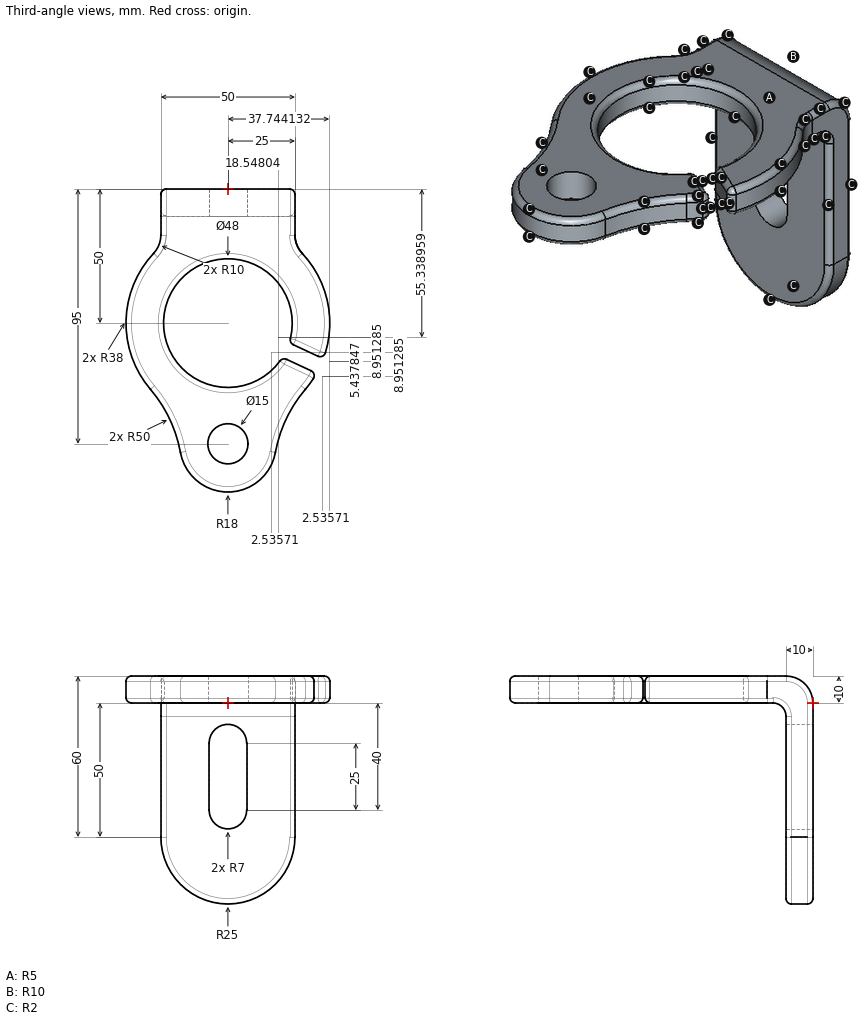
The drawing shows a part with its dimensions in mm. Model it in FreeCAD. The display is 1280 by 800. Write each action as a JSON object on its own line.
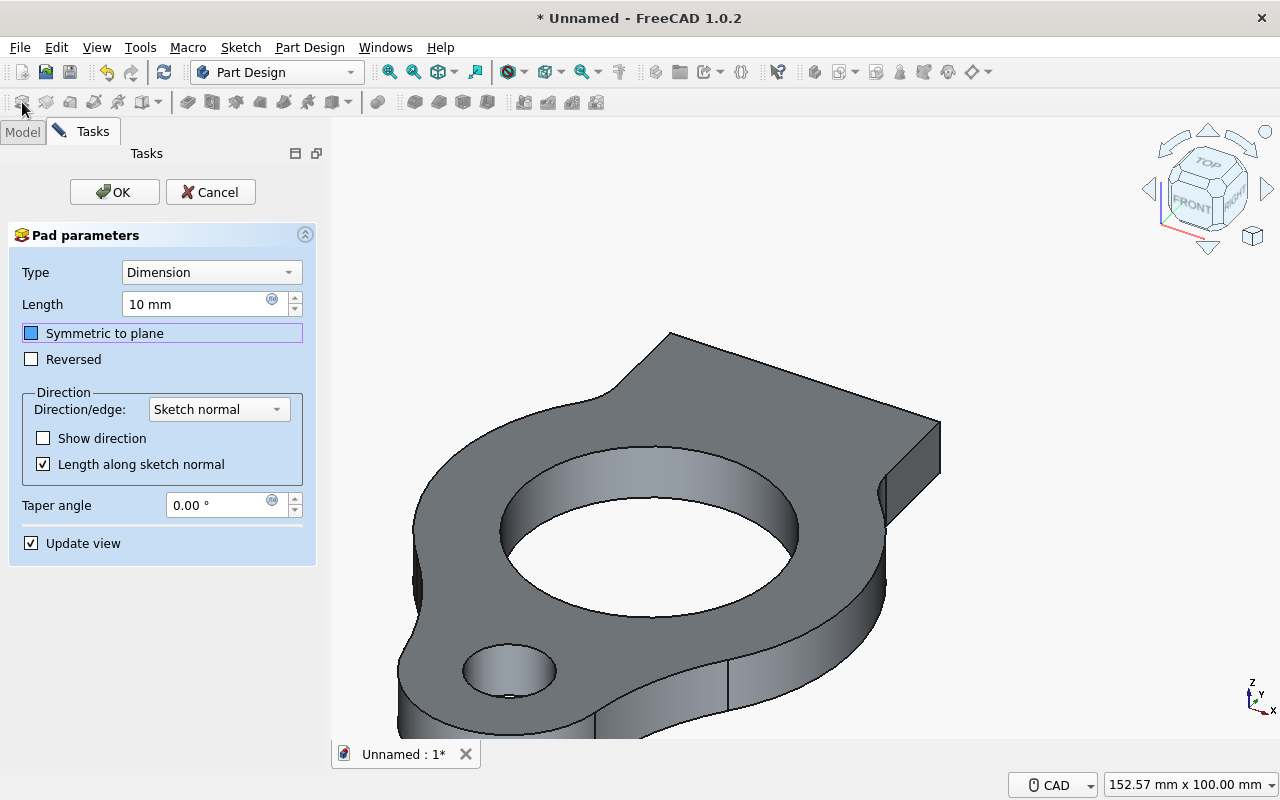
{"action": "left_click", "coordinate": [115, 192]}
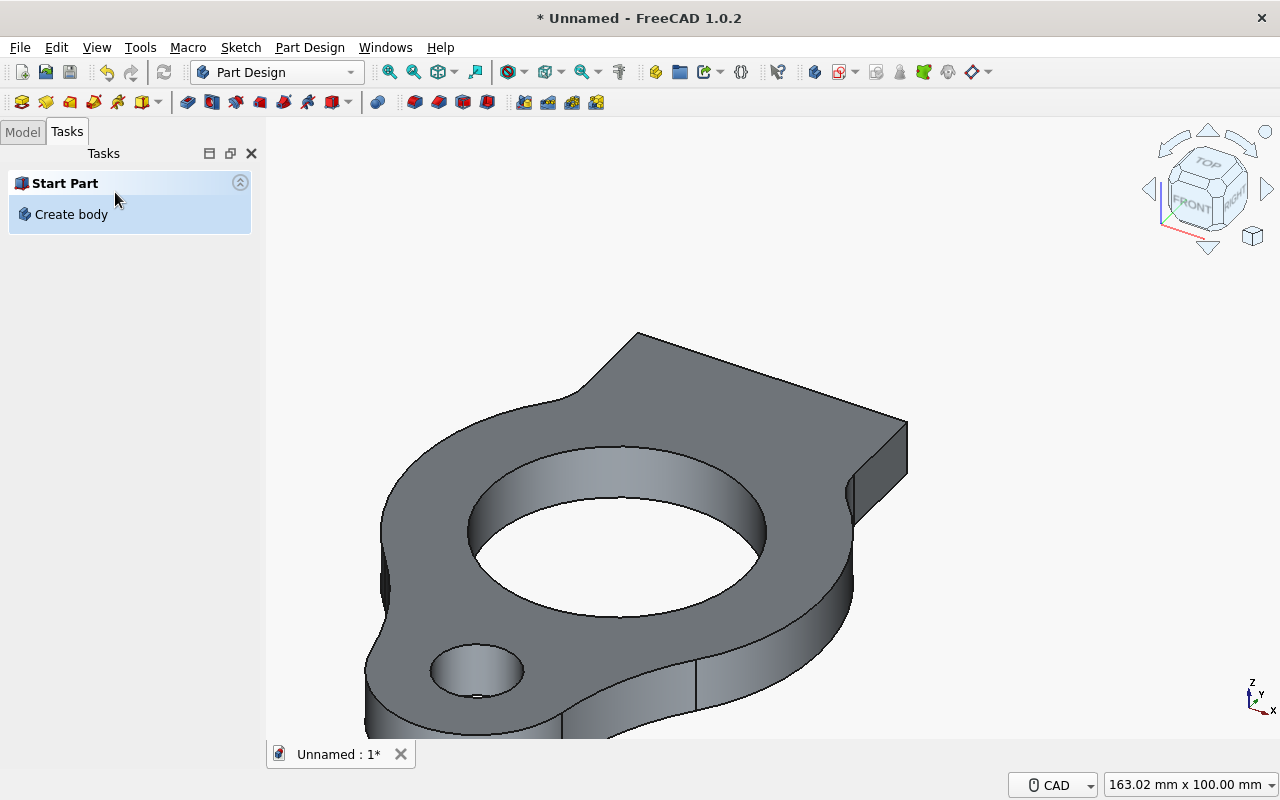
{"action": "left_click", "coordinate": [390, 72]}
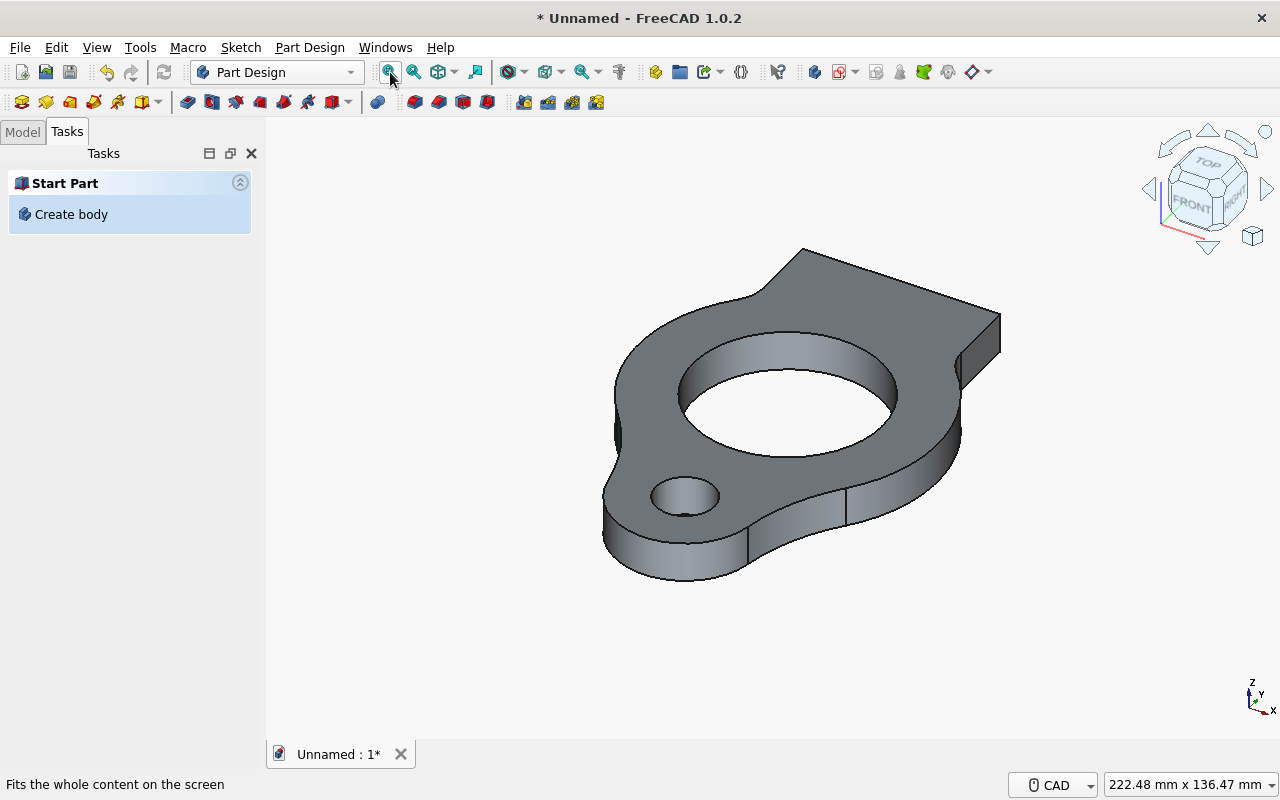
{"action": "key", "text": "4"}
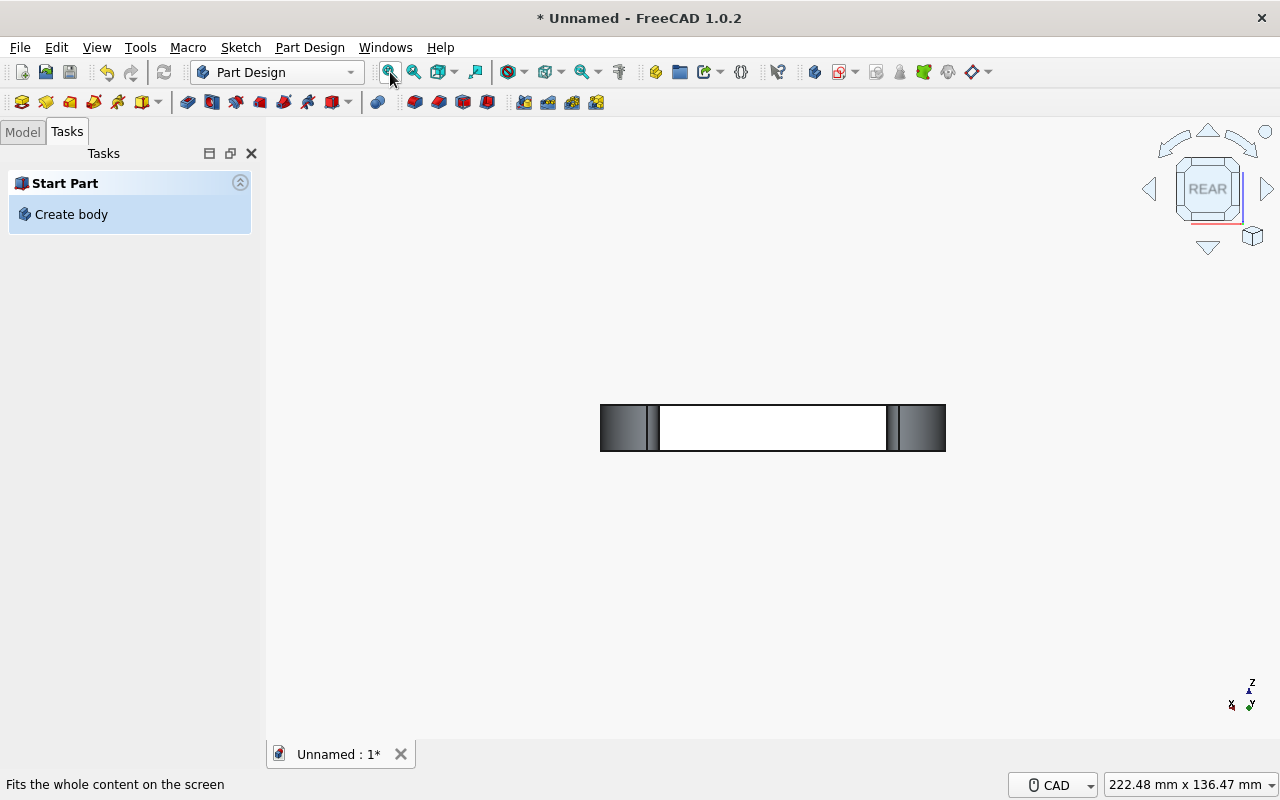
{"action": "left_click", "coordinate": [390, 72]}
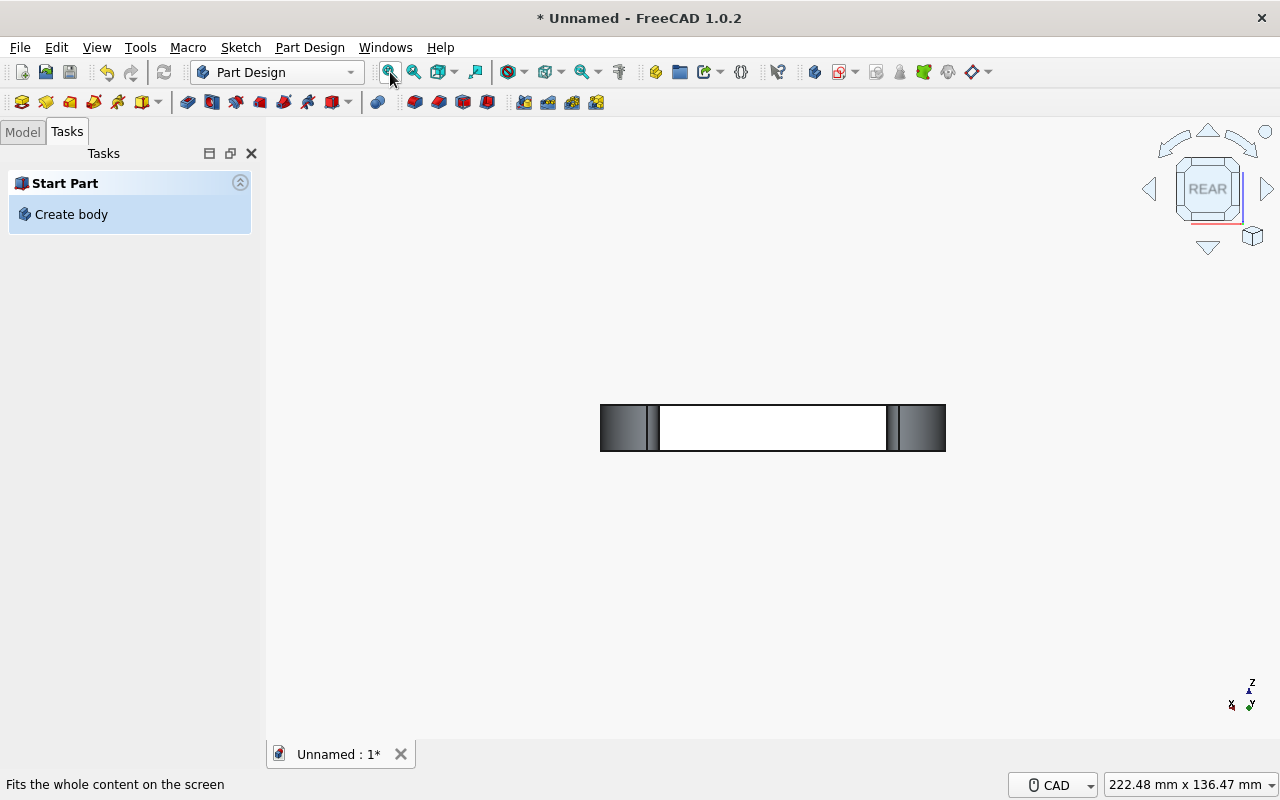
{"action": "left_click", "coordinate": [708, 427]}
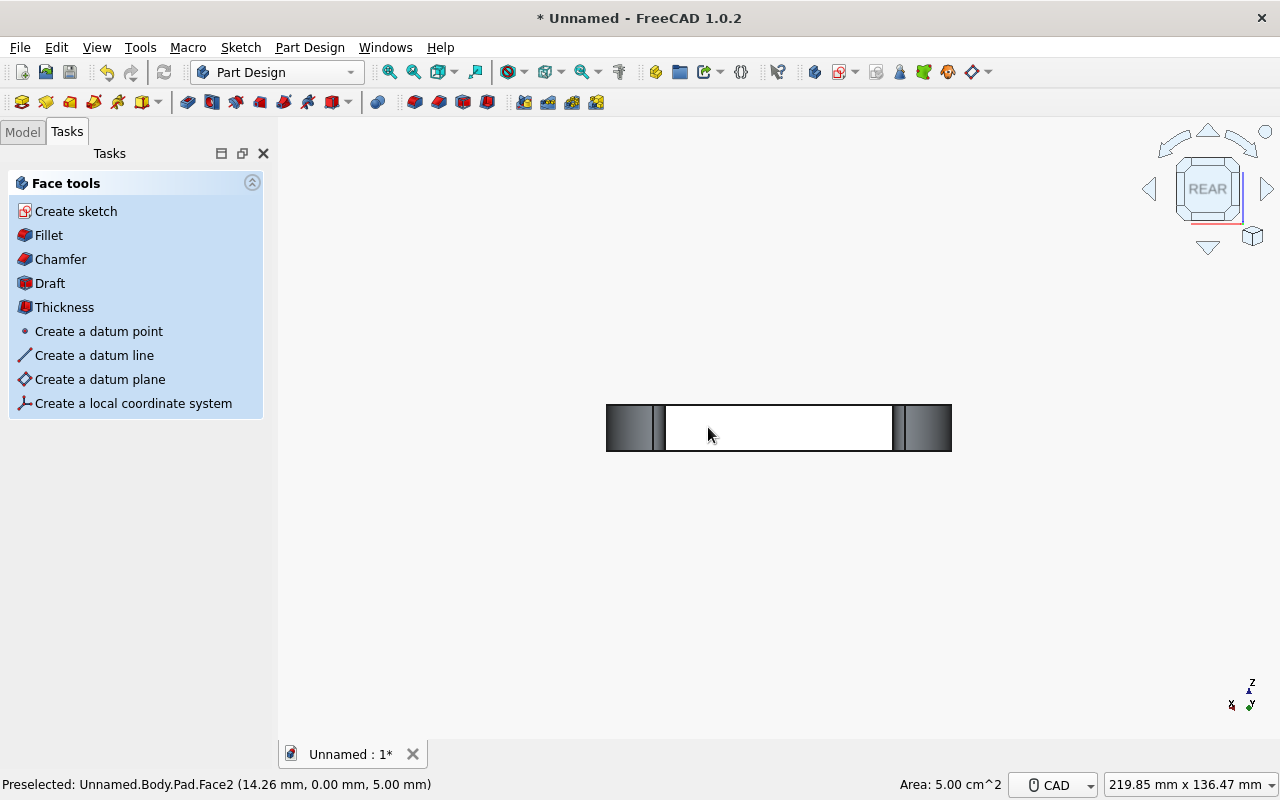
{"action": "left_click", "coordinate": [840, 72]}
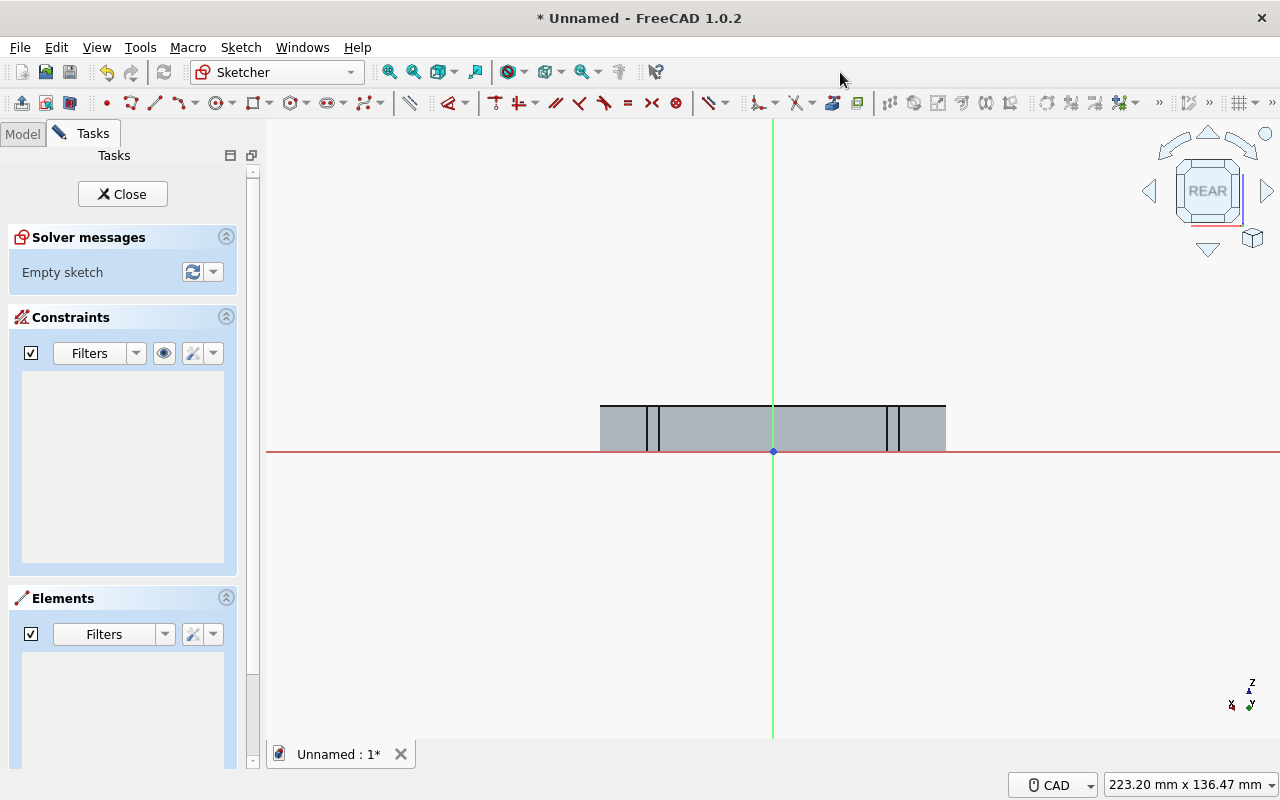
{"action": "scroll", "coordinate": [395, 147], "scroll_direction": "down", "scroll_amount": 1}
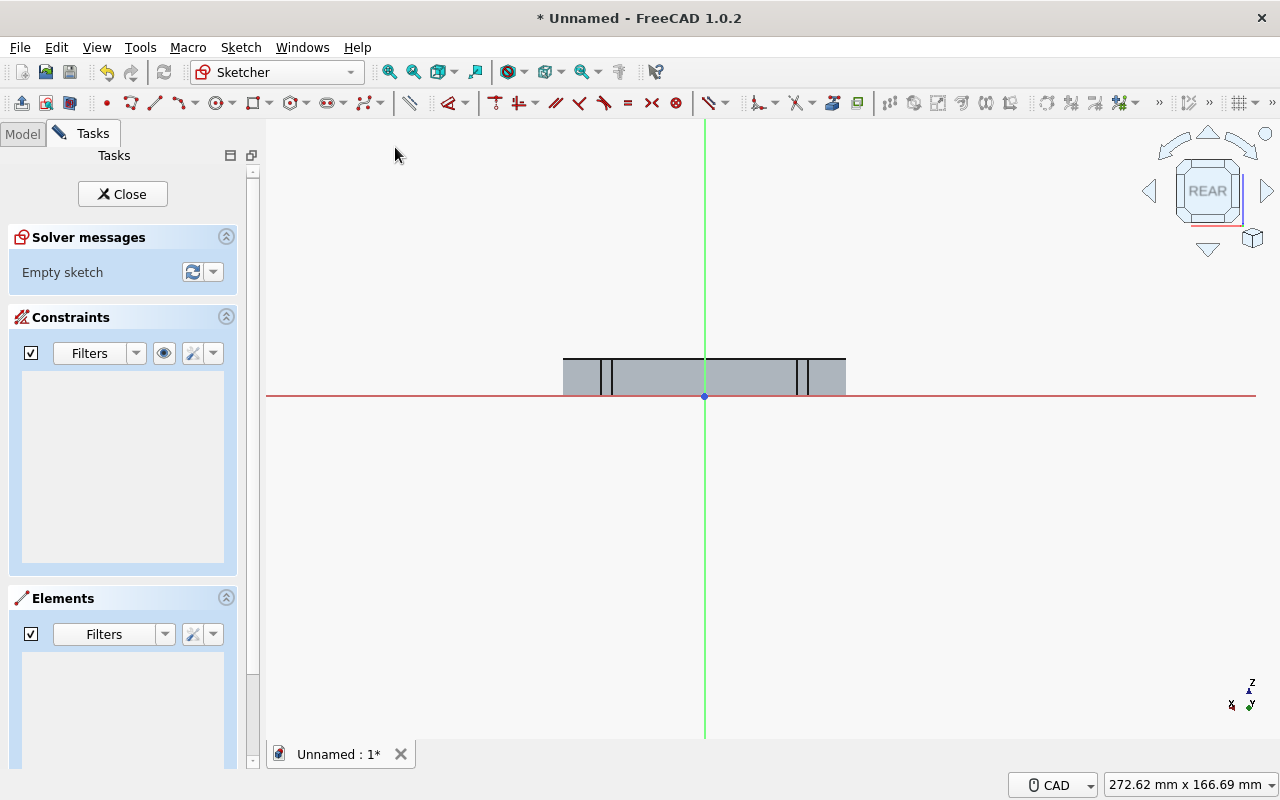
{"action": "left_click", "coordinate": [132, 104]}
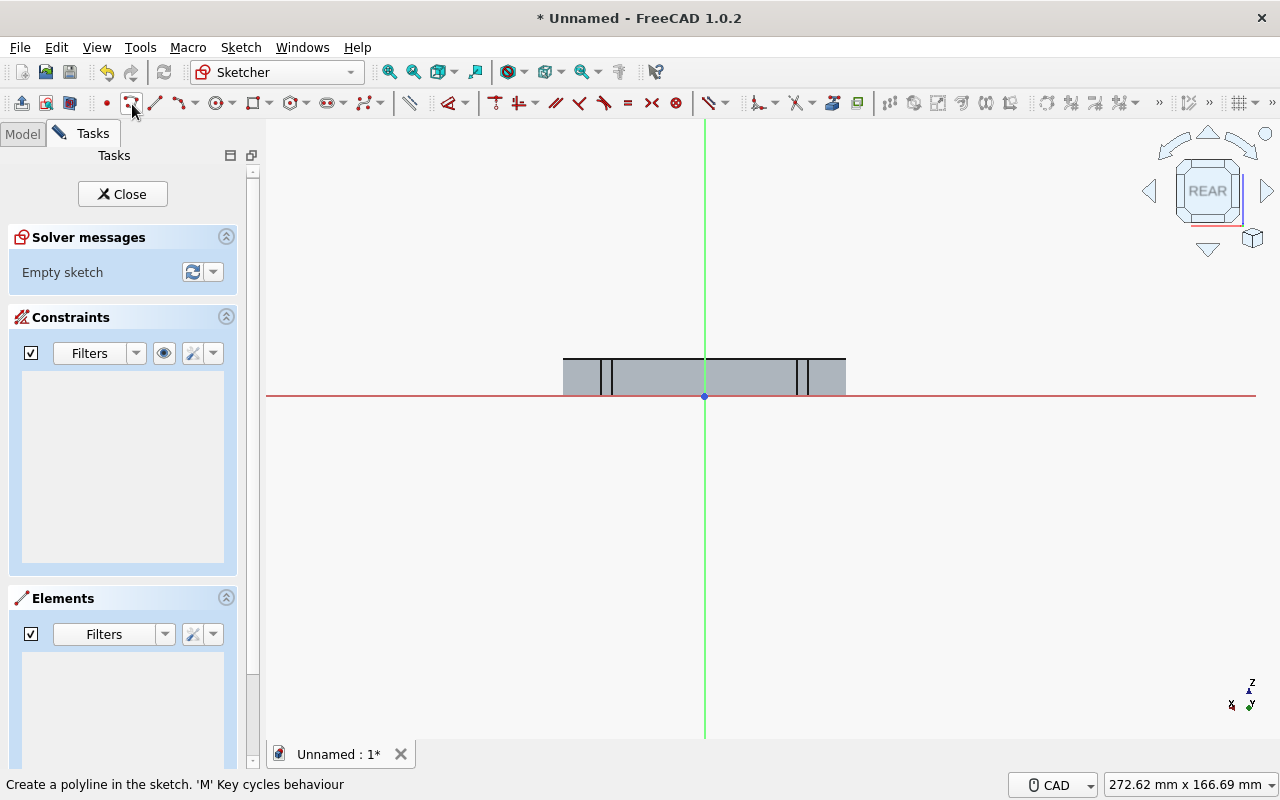
{"action": "left_click", "coordinate": [797, 582]}
{"action": "left_click", "coordinate": [797, 359]}
{"action": "left_click", "coordinate": [612, 359]}
{"action": "left_click", "coordinate": [612, 582]}
{"action": "right_click", "coordinate": [612, 582]}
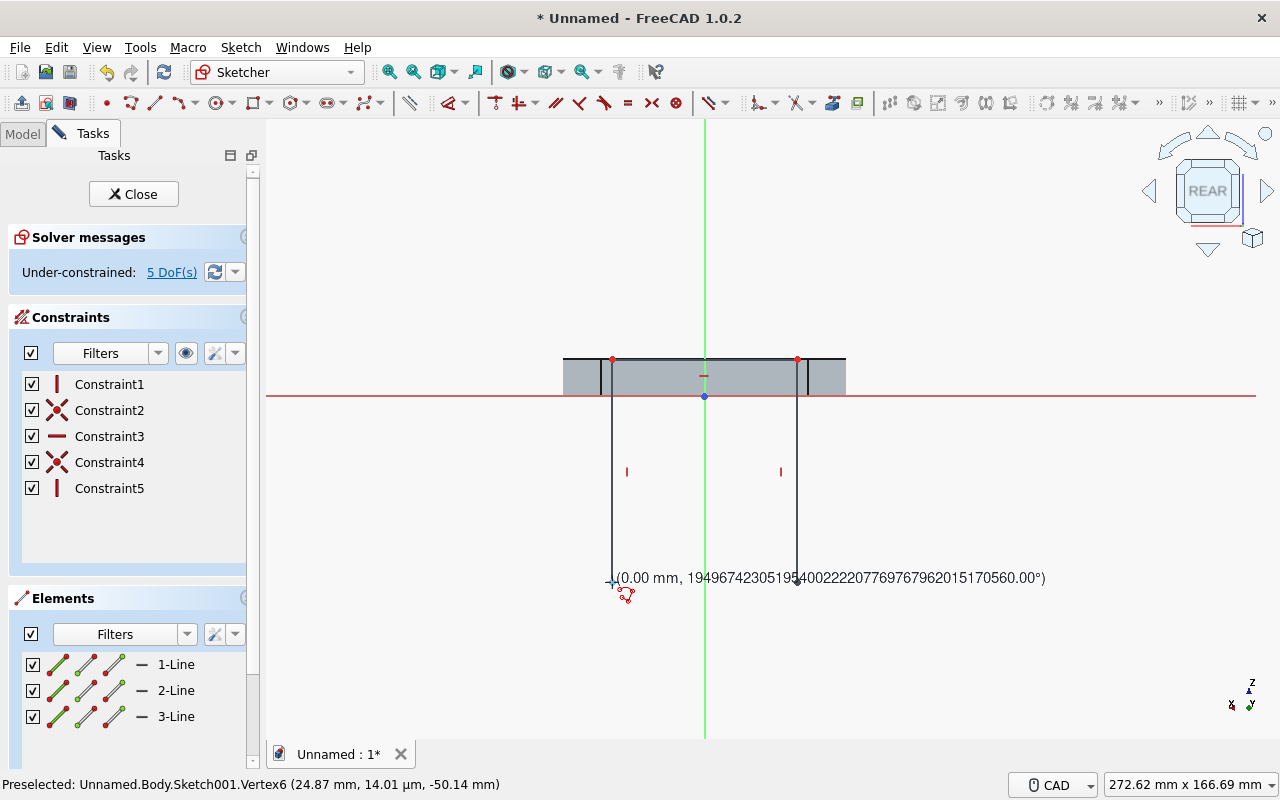
{"action": "left_click", "coordinate": [180, 104]}